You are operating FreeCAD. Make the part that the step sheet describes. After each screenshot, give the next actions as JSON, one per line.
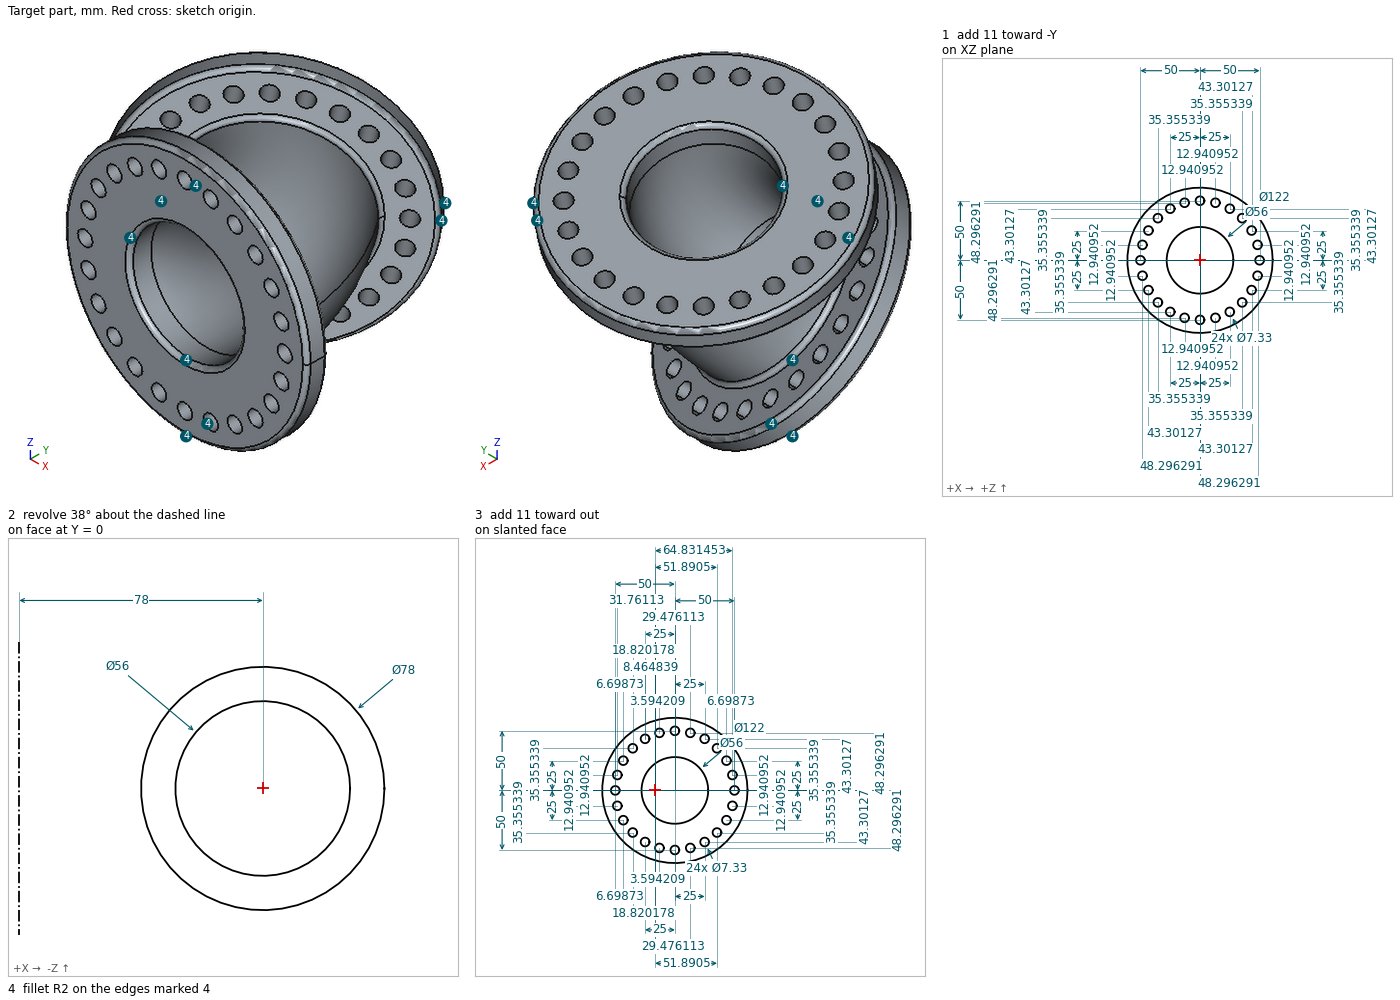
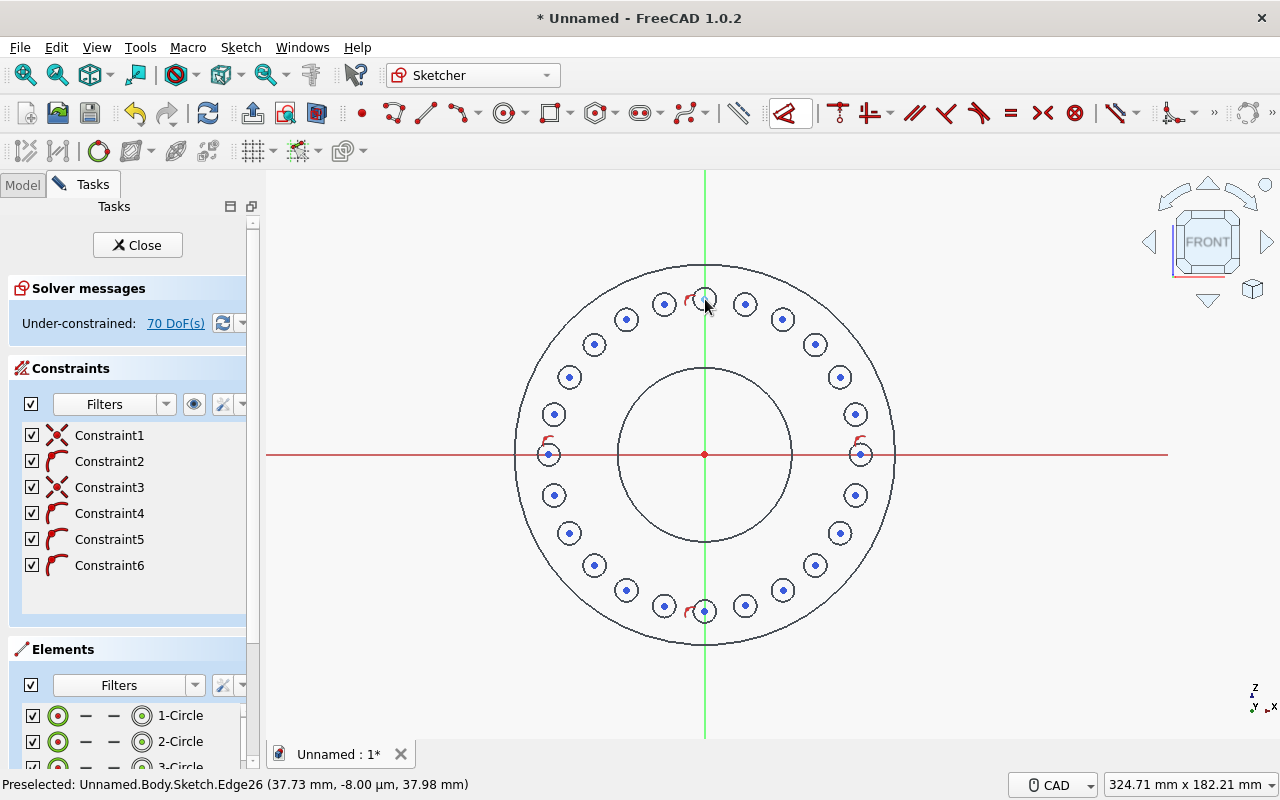
{"action": "left_click", "coordinate": [603, 558]}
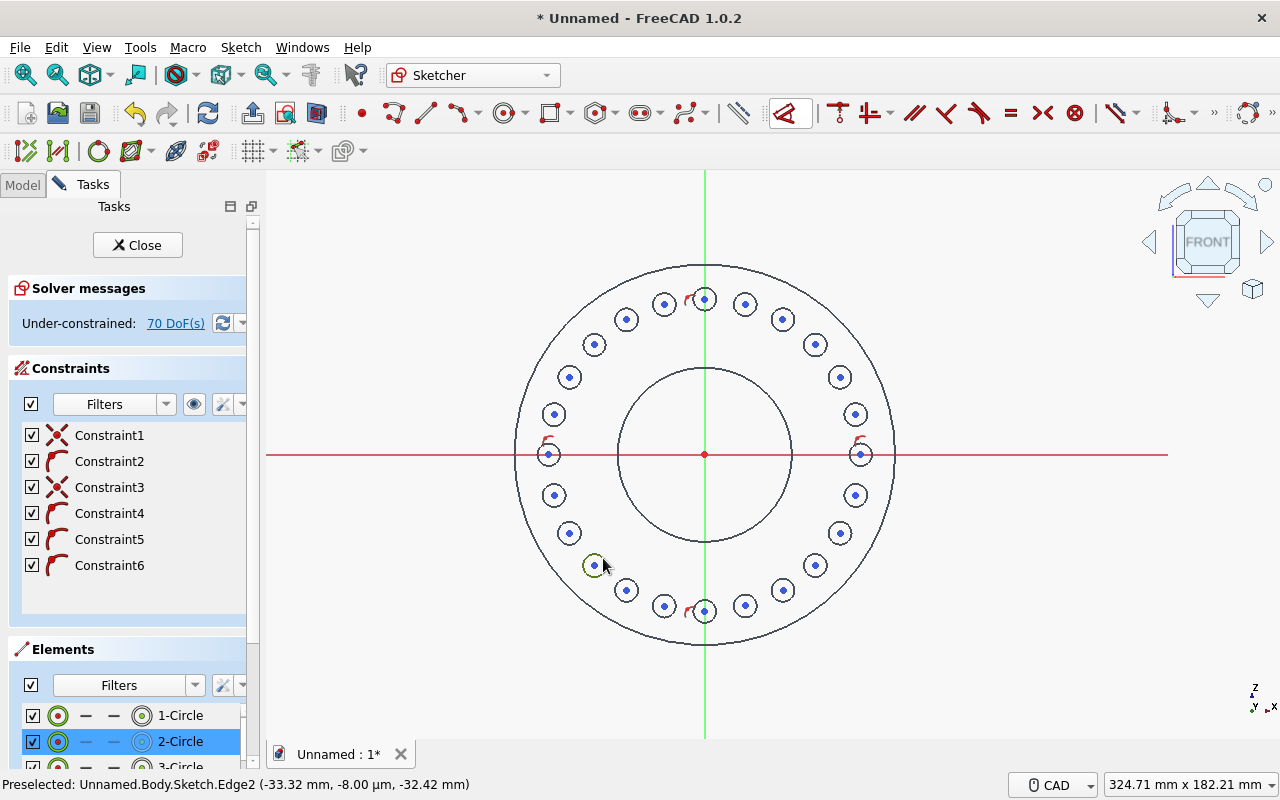
{"action": "left_click", "coordinate": [578, 525]}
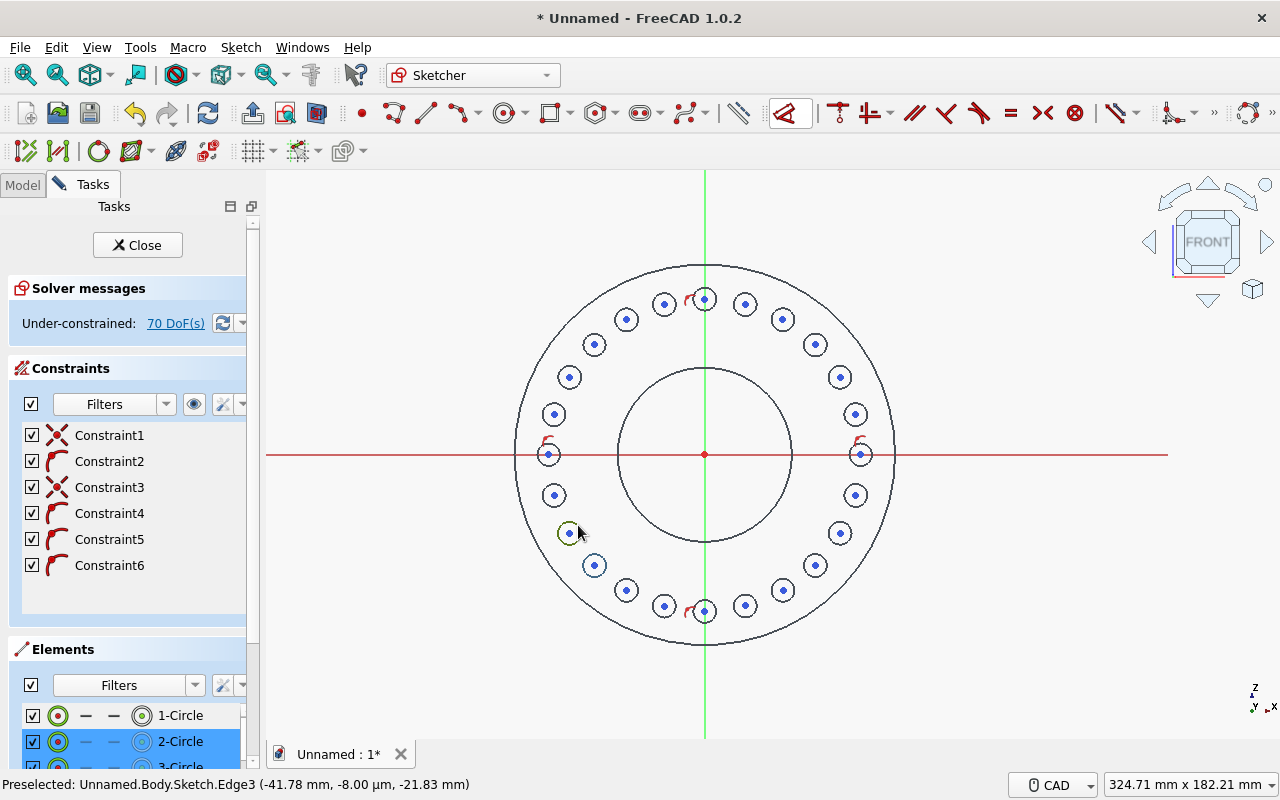
{"action": "left_click", "coordinate": [562, 487]}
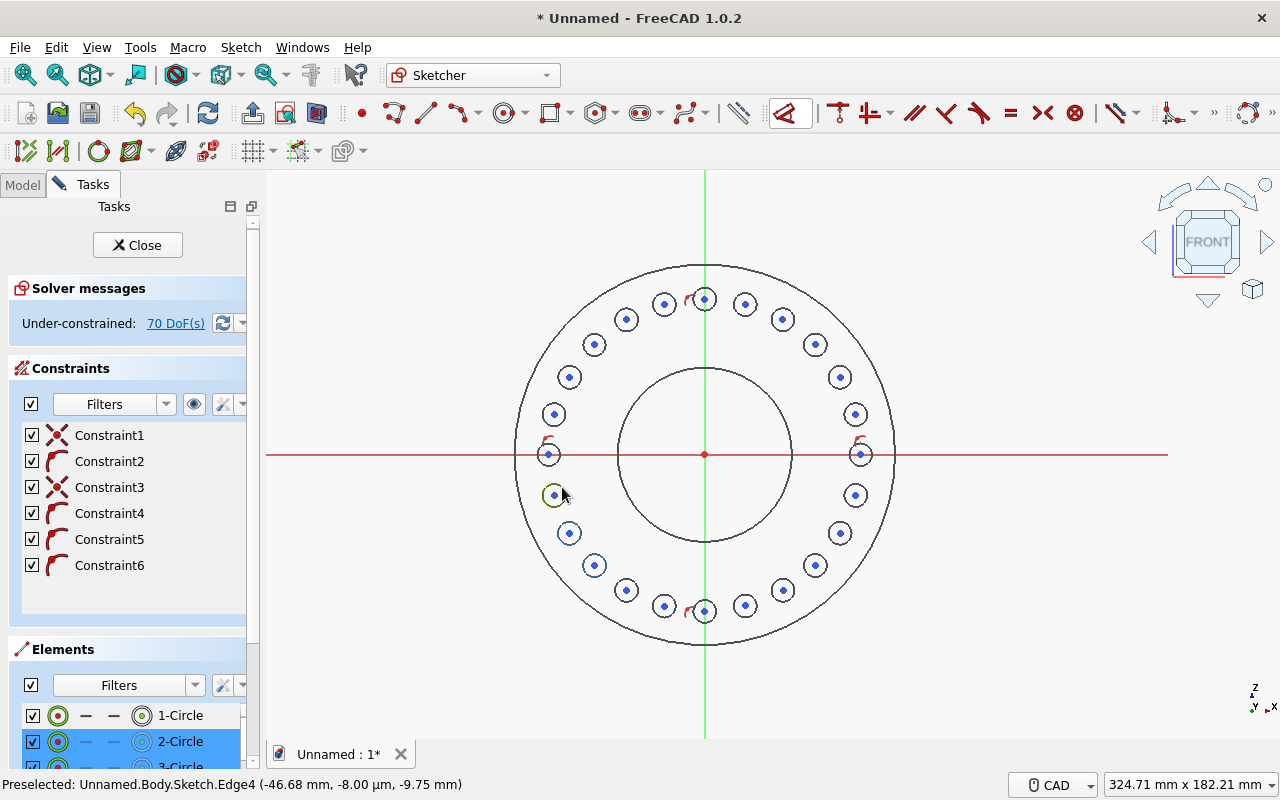
{"action": "left_click", "coordinate": [635, 582]}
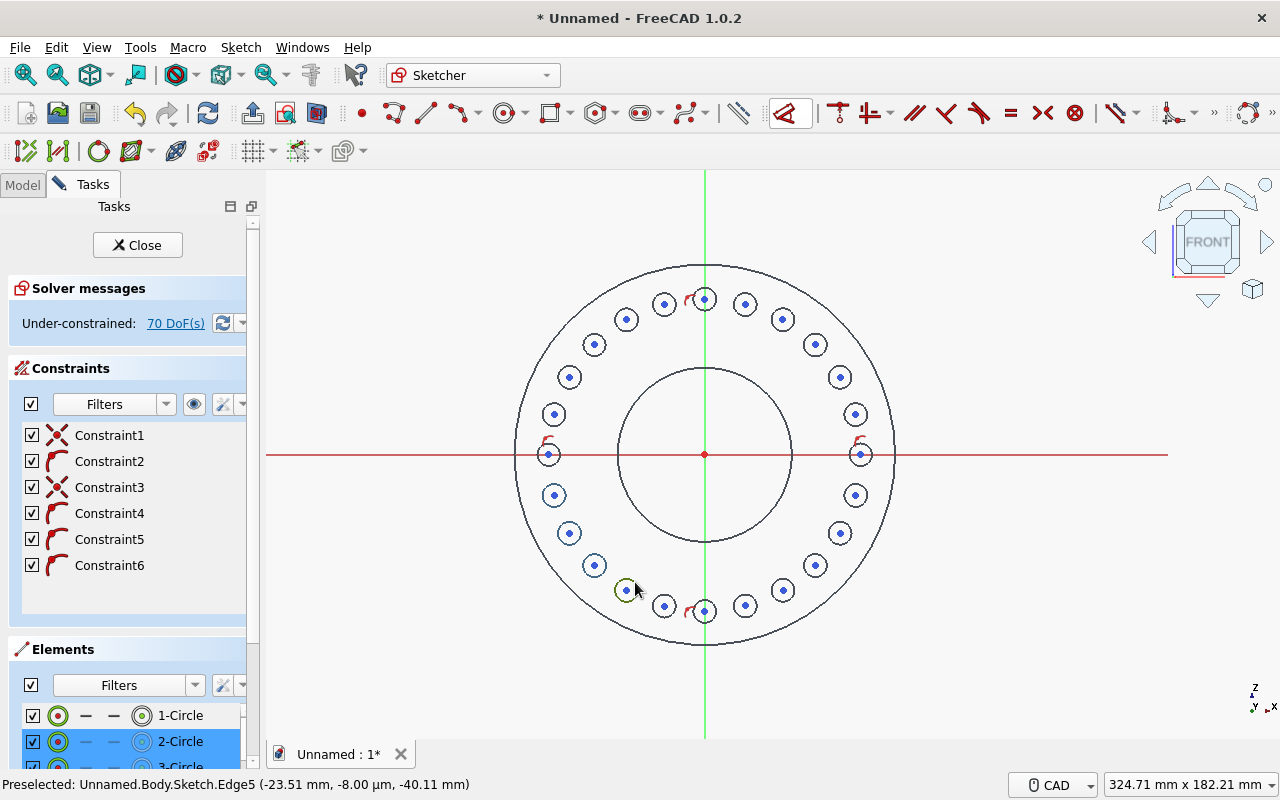
{"action": "left_click", "coordinate": [672, 598]}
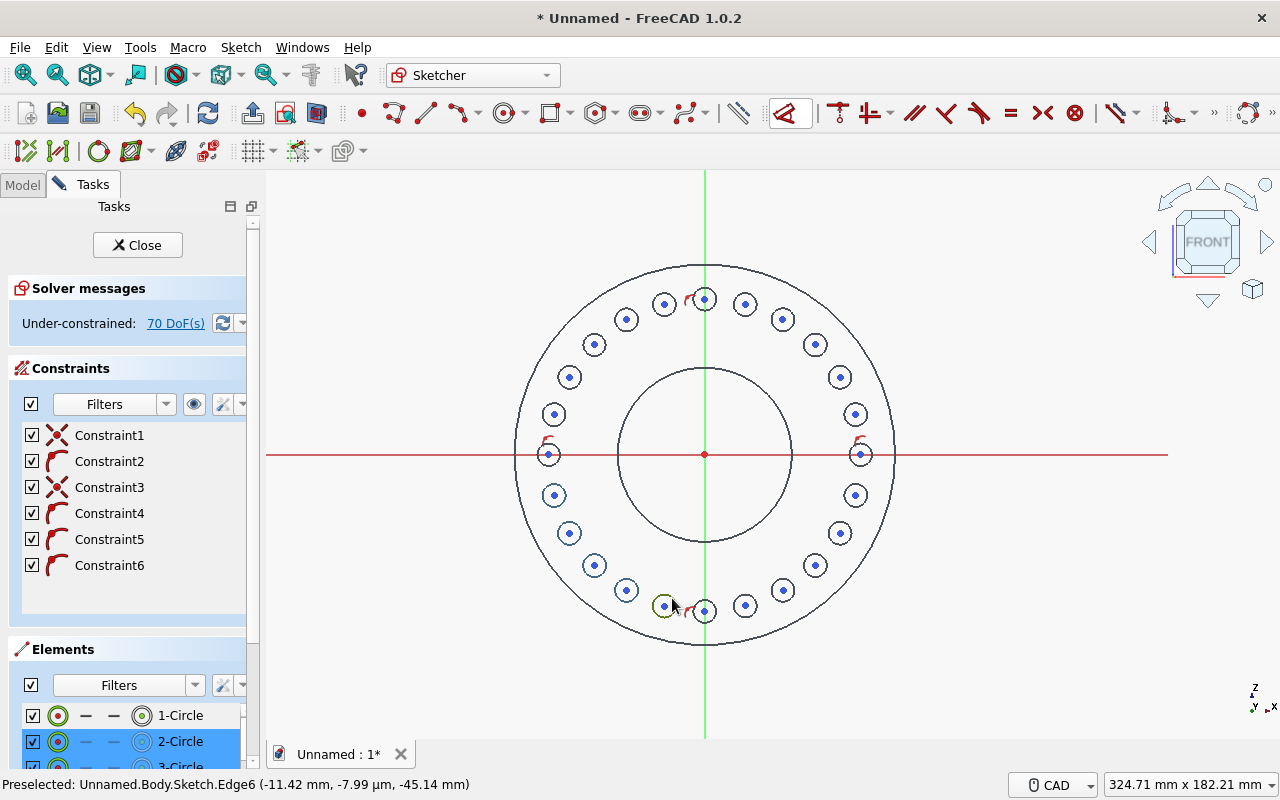
{"action": "left_click", "coordinate": [705, 600]}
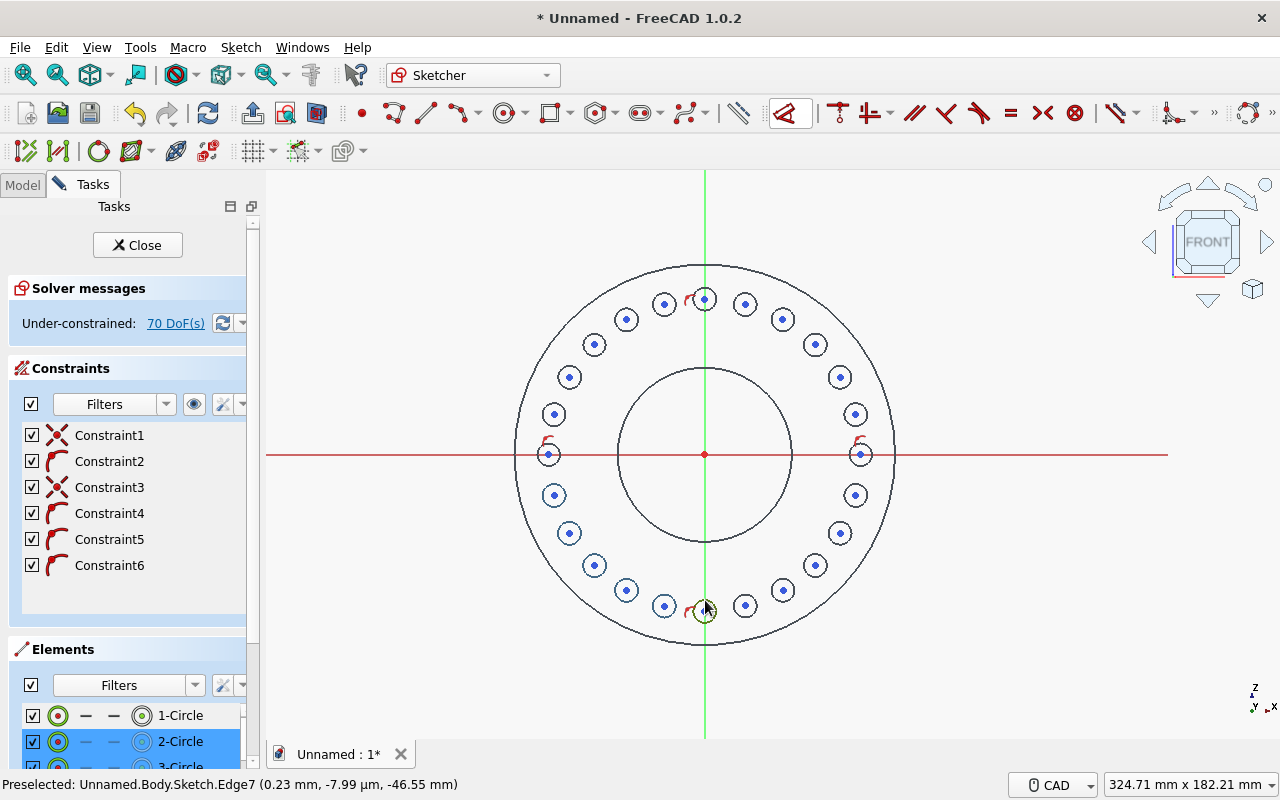
{"action": "scroll", "coordinate": [549, 444], "scroll_direction": "up", "scroll_amount": 2}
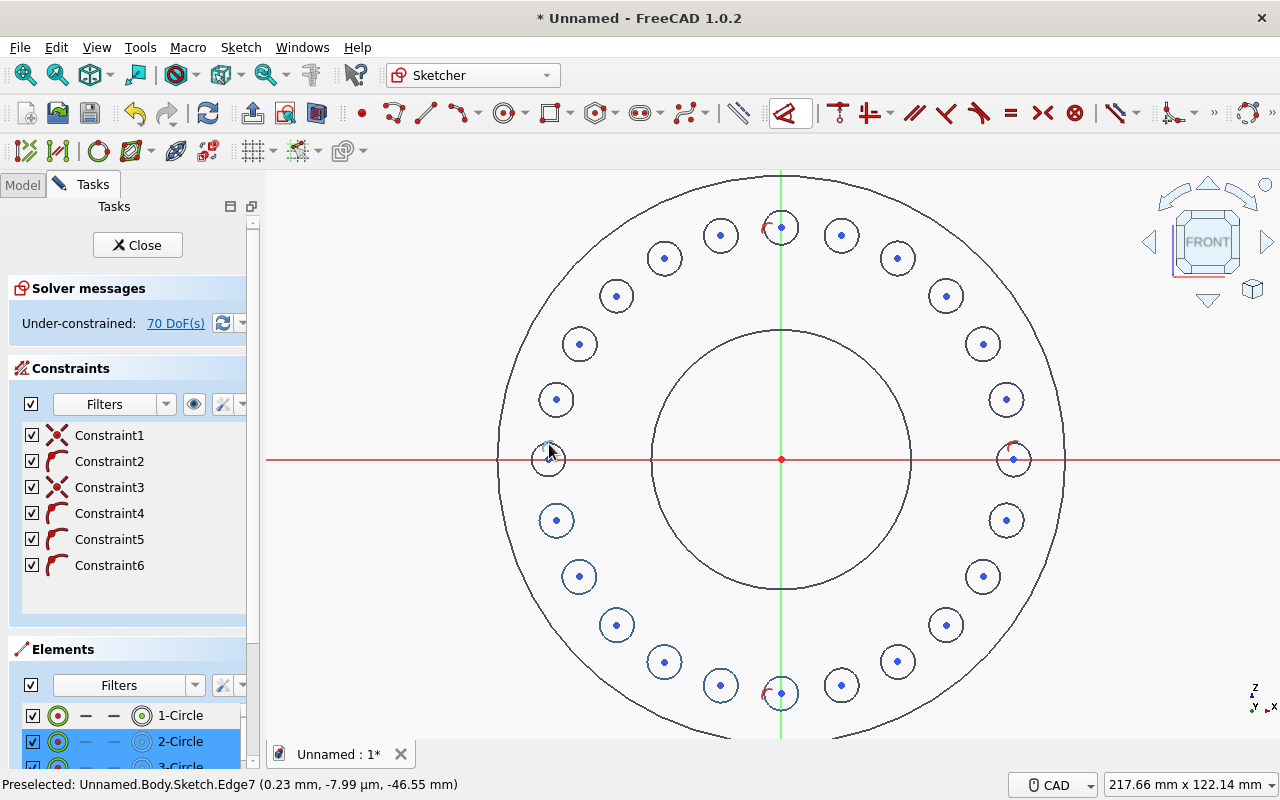
{"action": "left_click", "coordinate": [532, 459]}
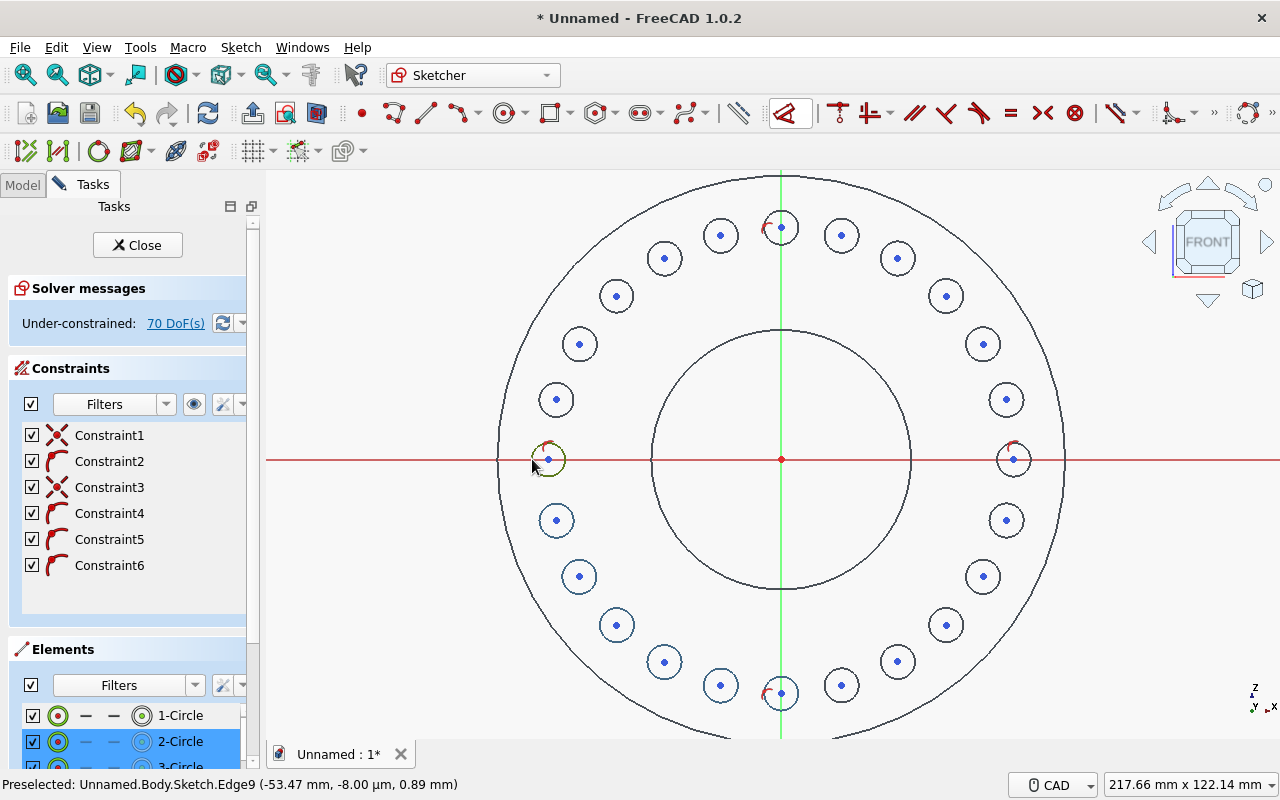
{"action": "left_click", "coordinate": [568, 388]}